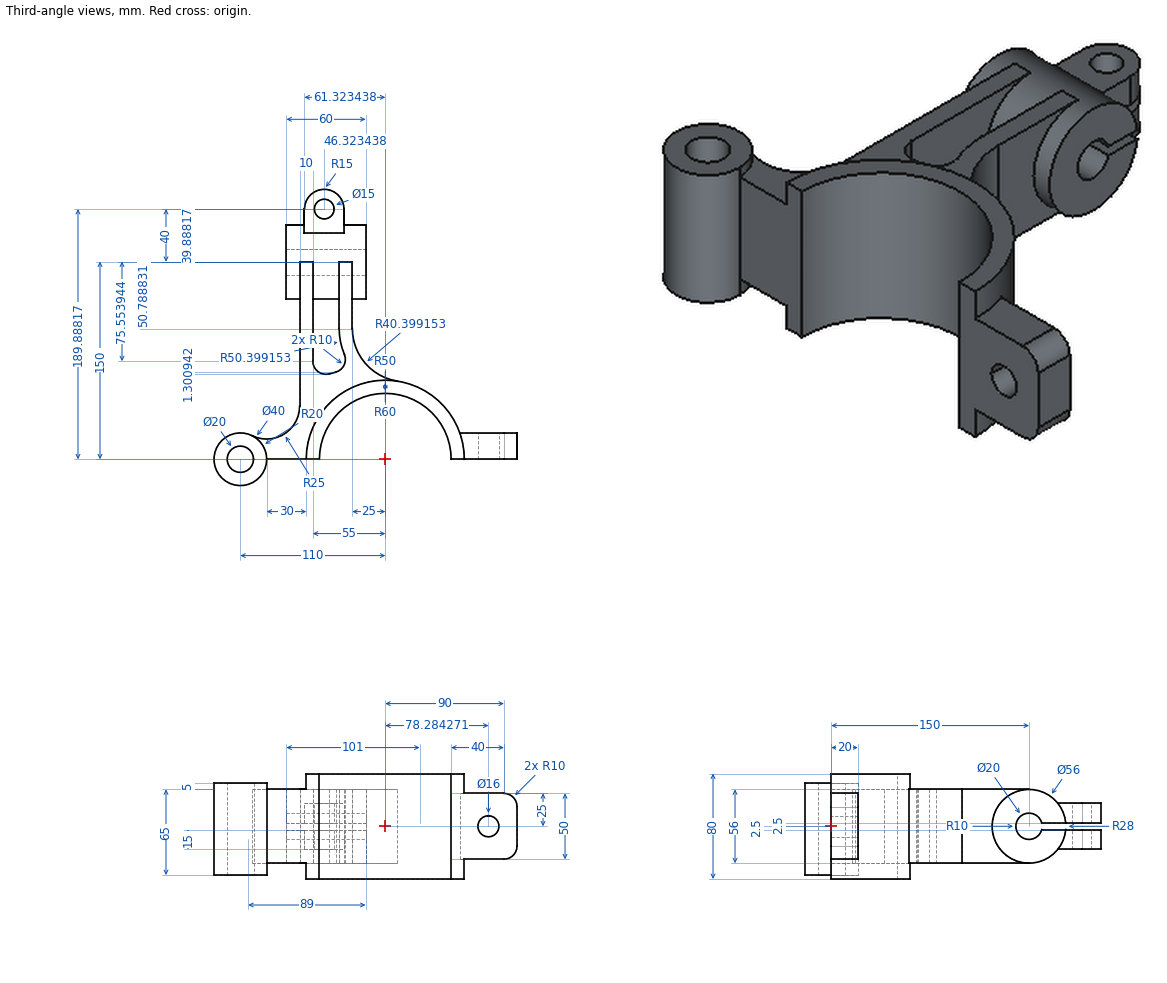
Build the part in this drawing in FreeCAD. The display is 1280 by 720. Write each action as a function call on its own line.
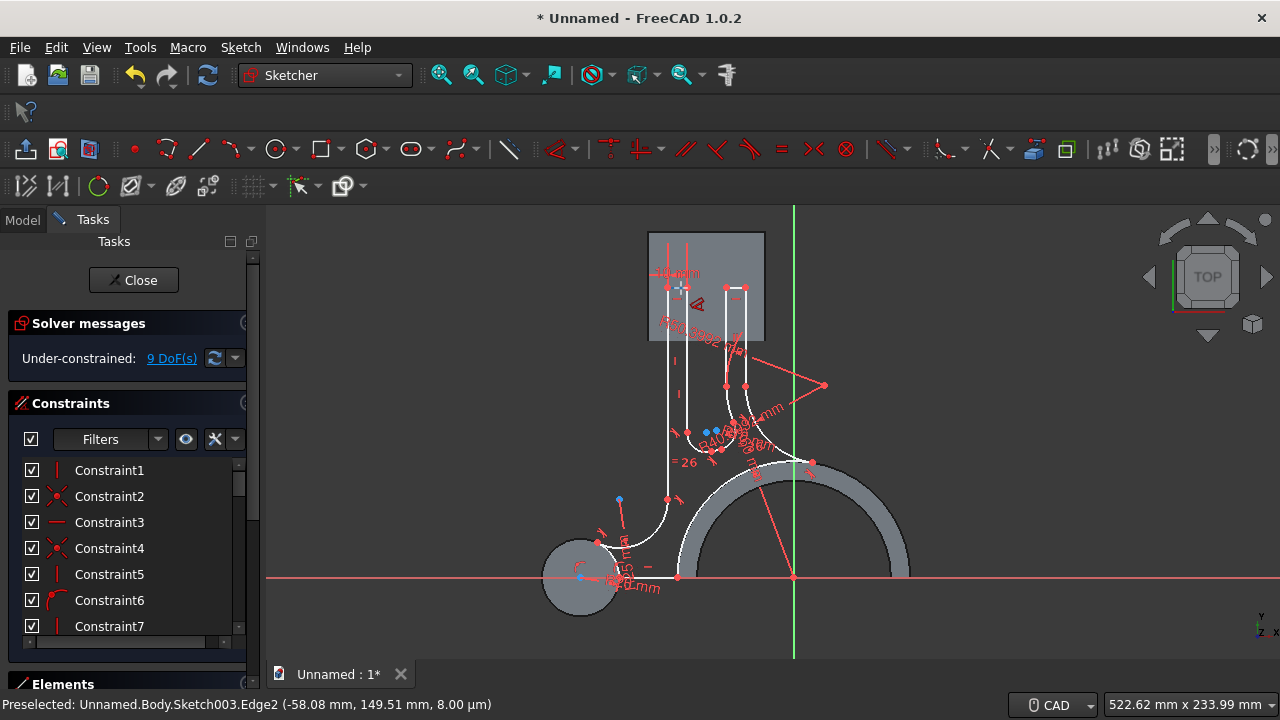
click(637, 578)
click(648, 612)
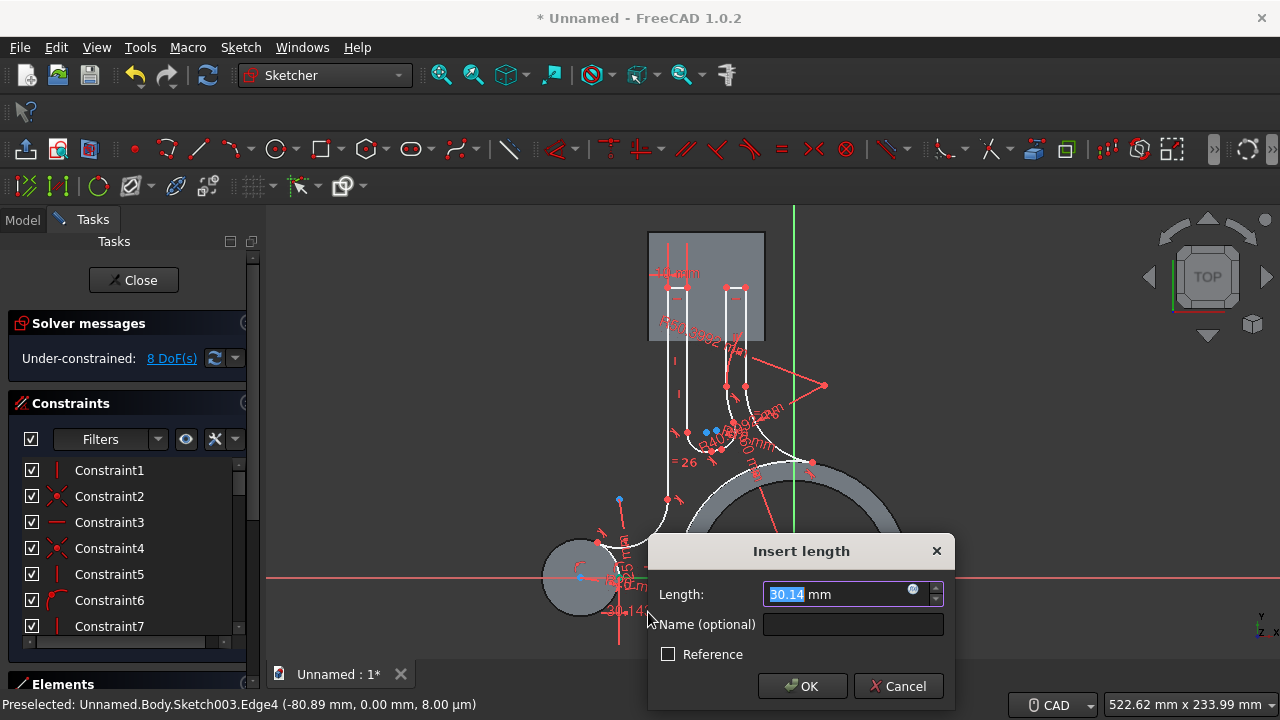
text(30)
key(Return)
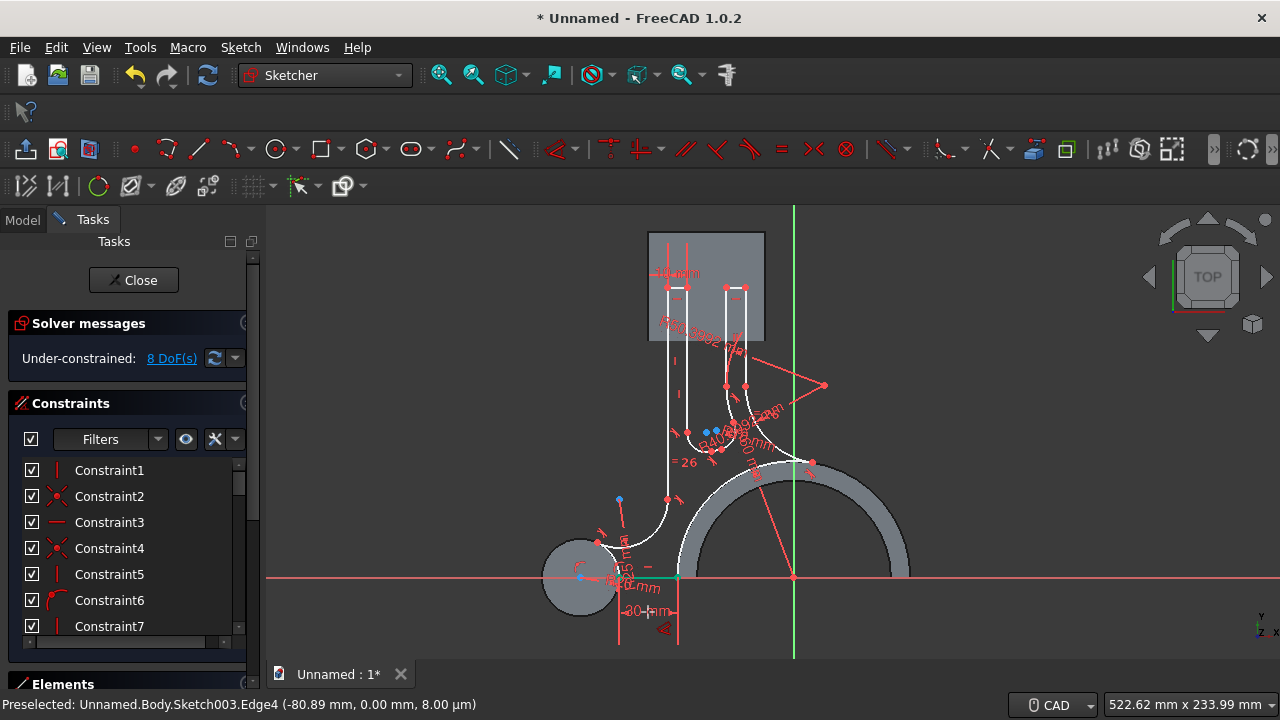
click(687, 433)
click(741, 612)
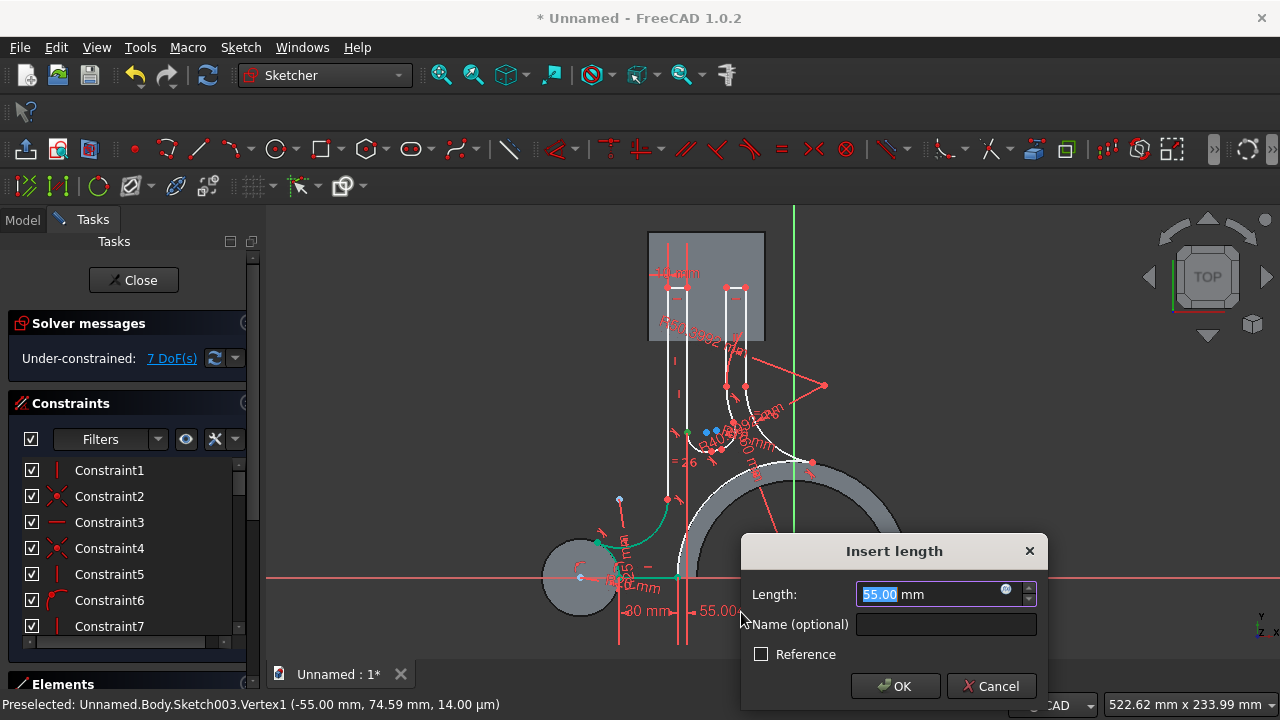
text(55)
key(Return)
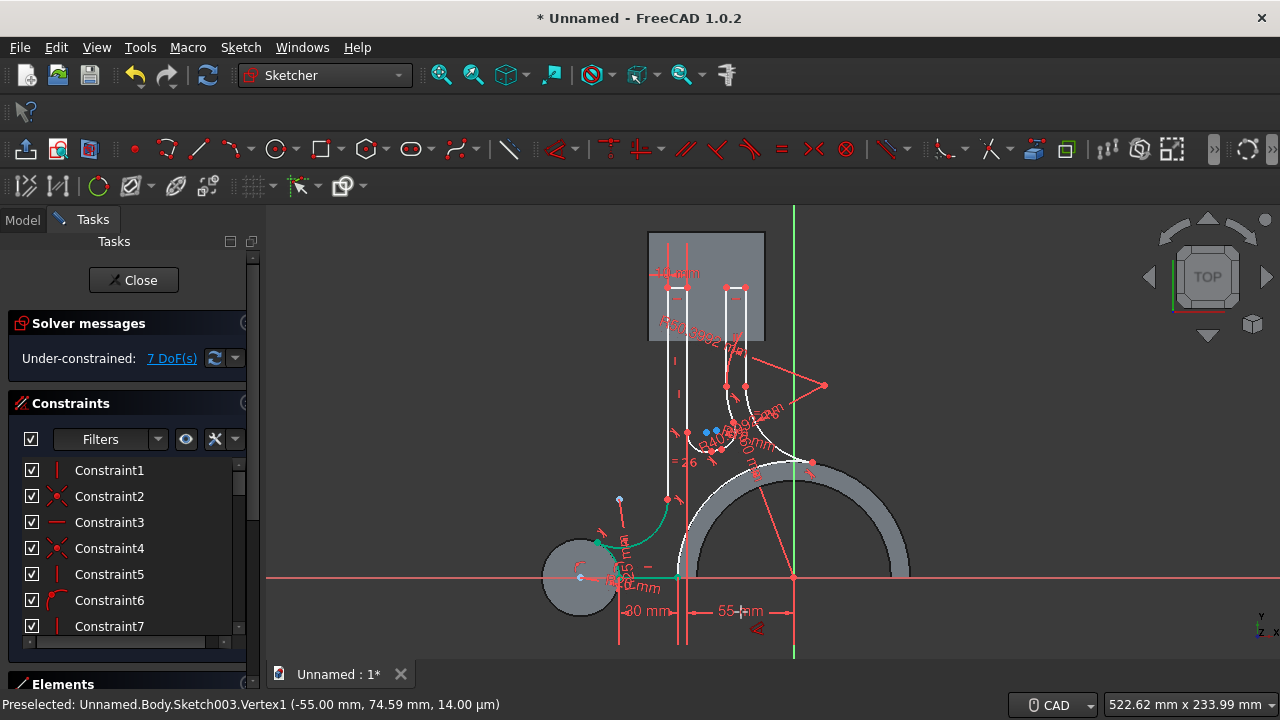
click(746, 386)
click(770, 304)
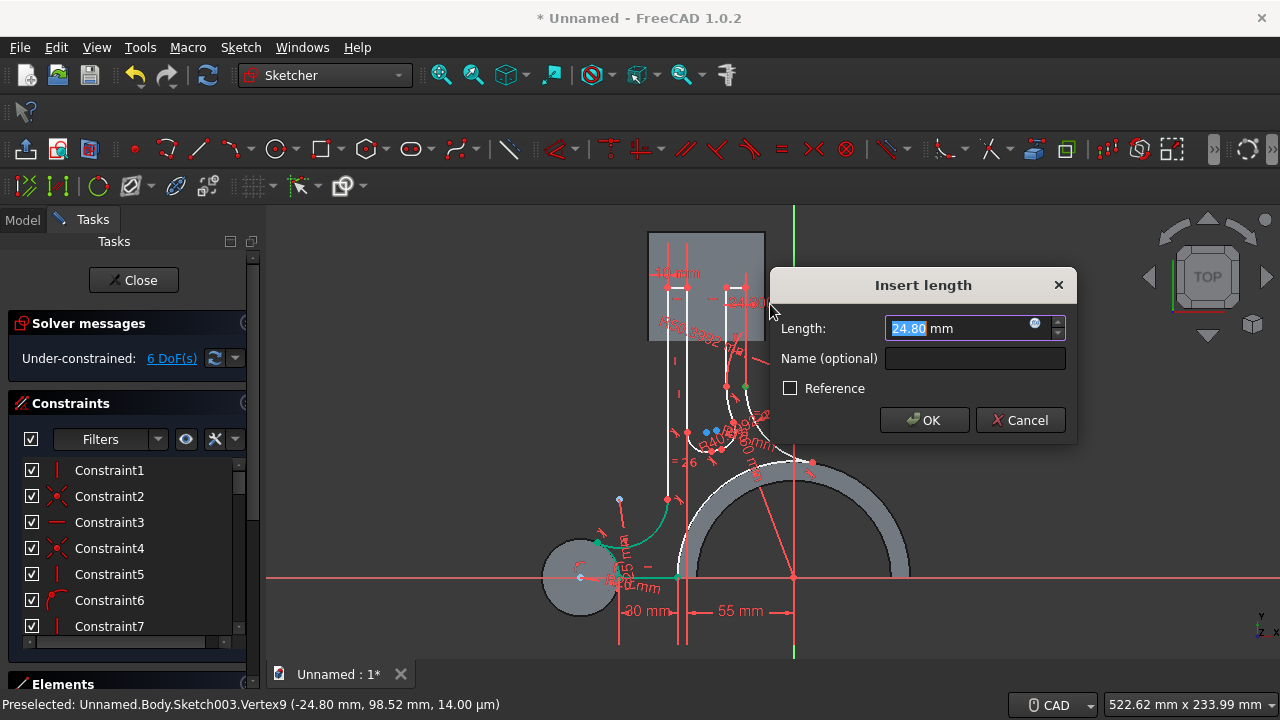
text(25)
key(Return)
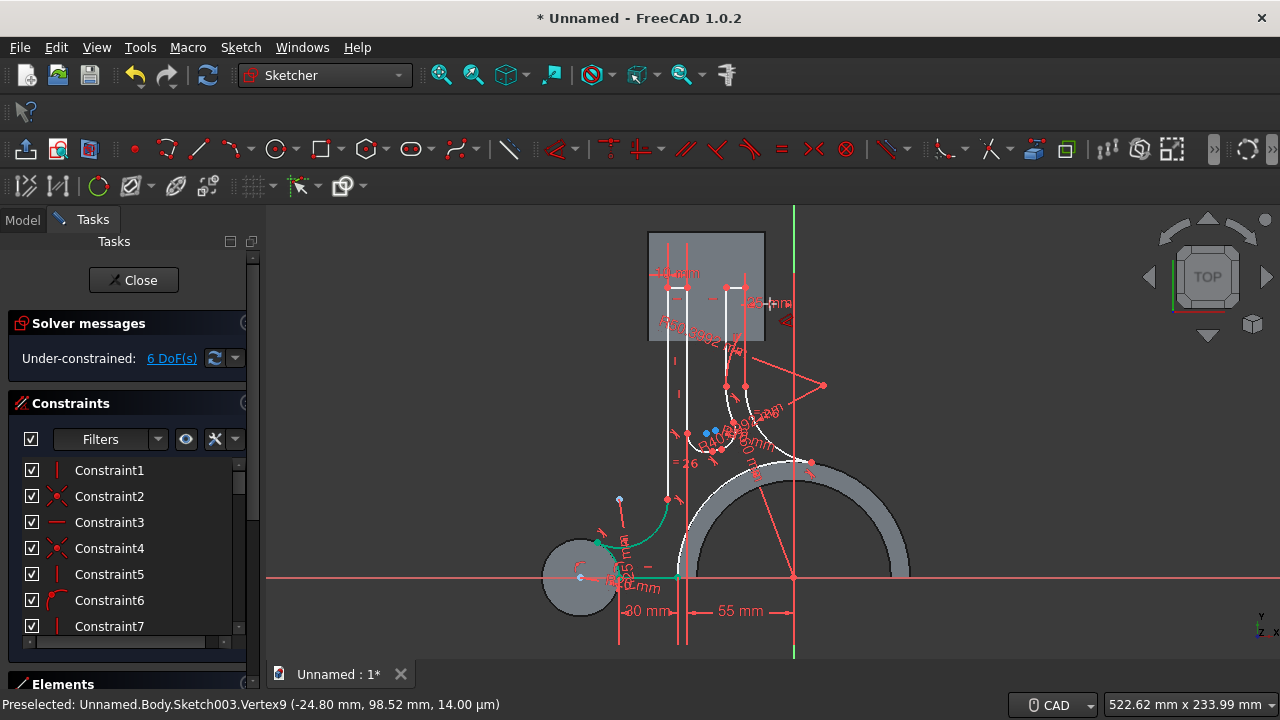
click(687, 288)
click(828, 433)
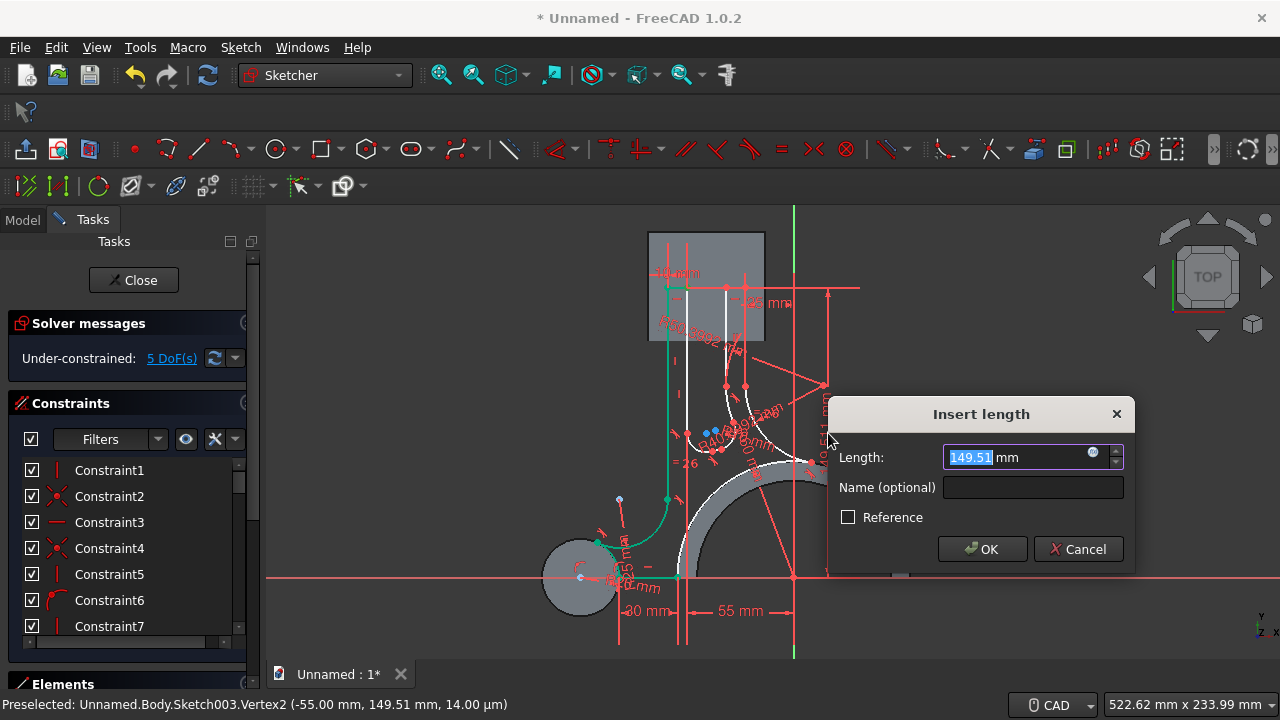
text(150)
key(Return)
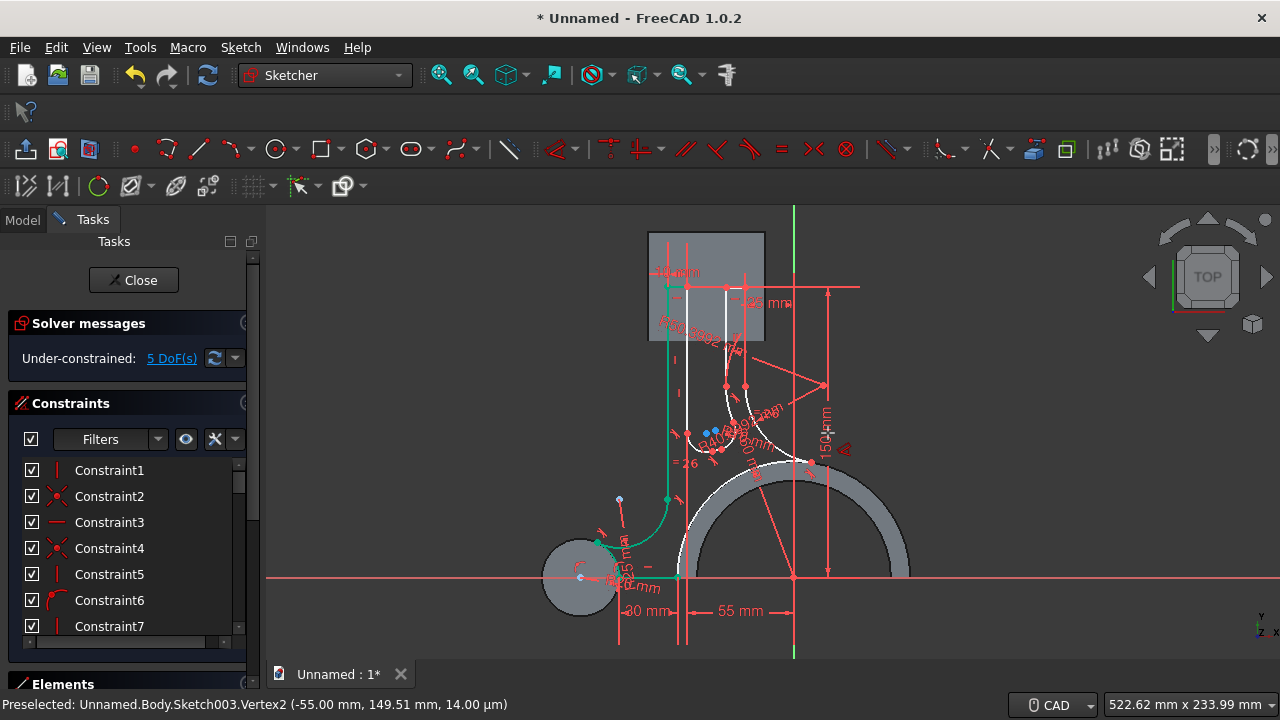
click(745, 288)
click(828, 366)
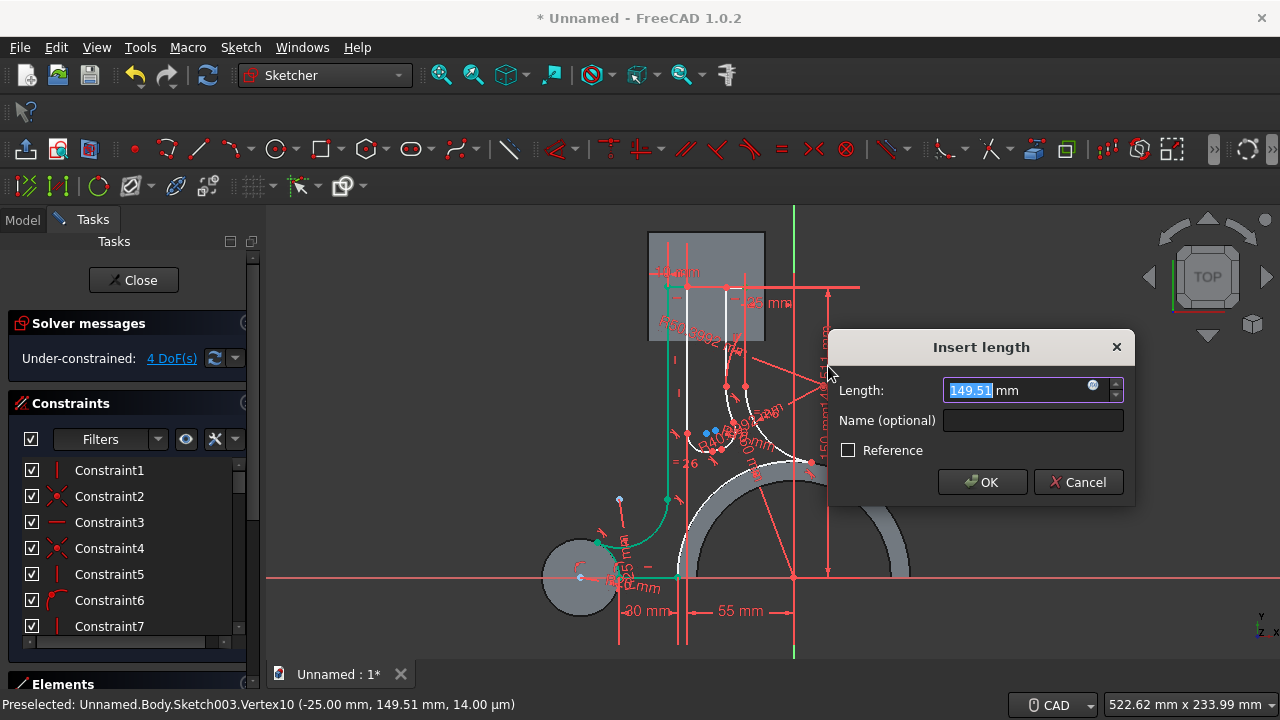
text(150)
key(Return)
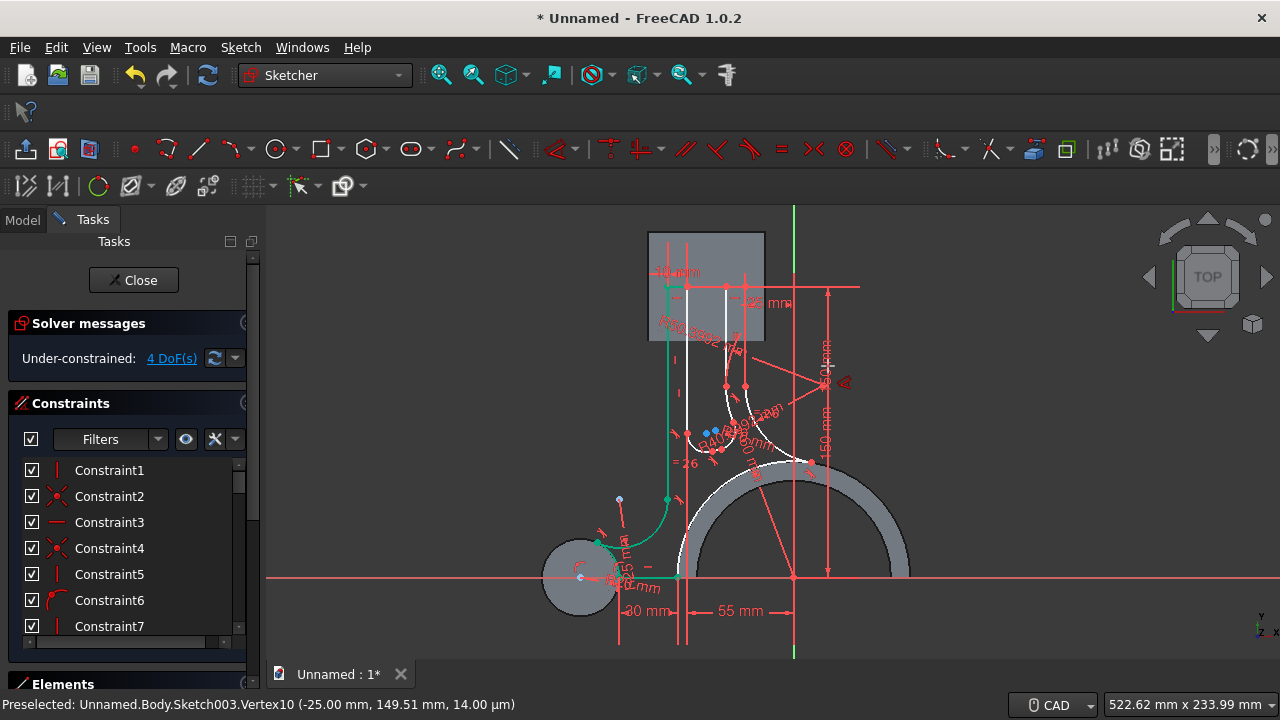
click(687, 389)
click(653, 360)